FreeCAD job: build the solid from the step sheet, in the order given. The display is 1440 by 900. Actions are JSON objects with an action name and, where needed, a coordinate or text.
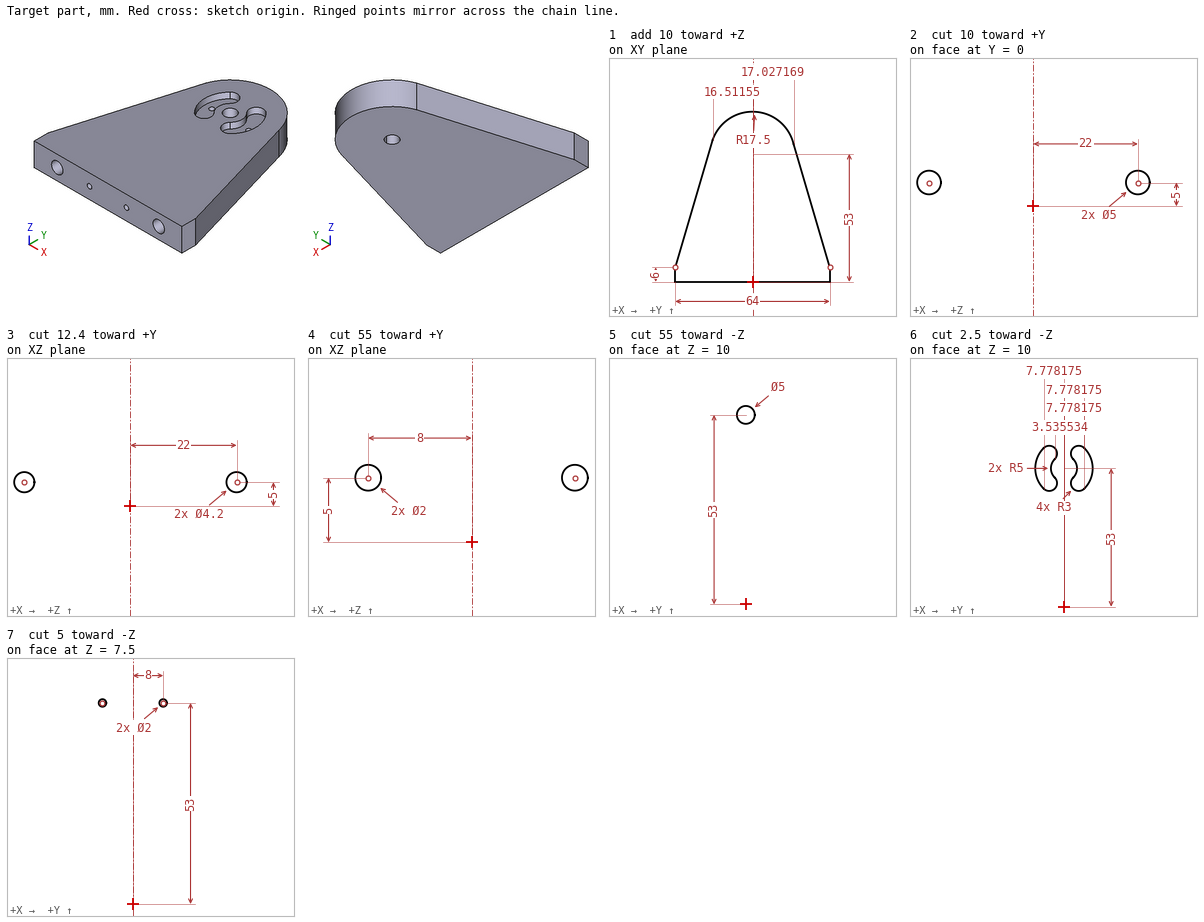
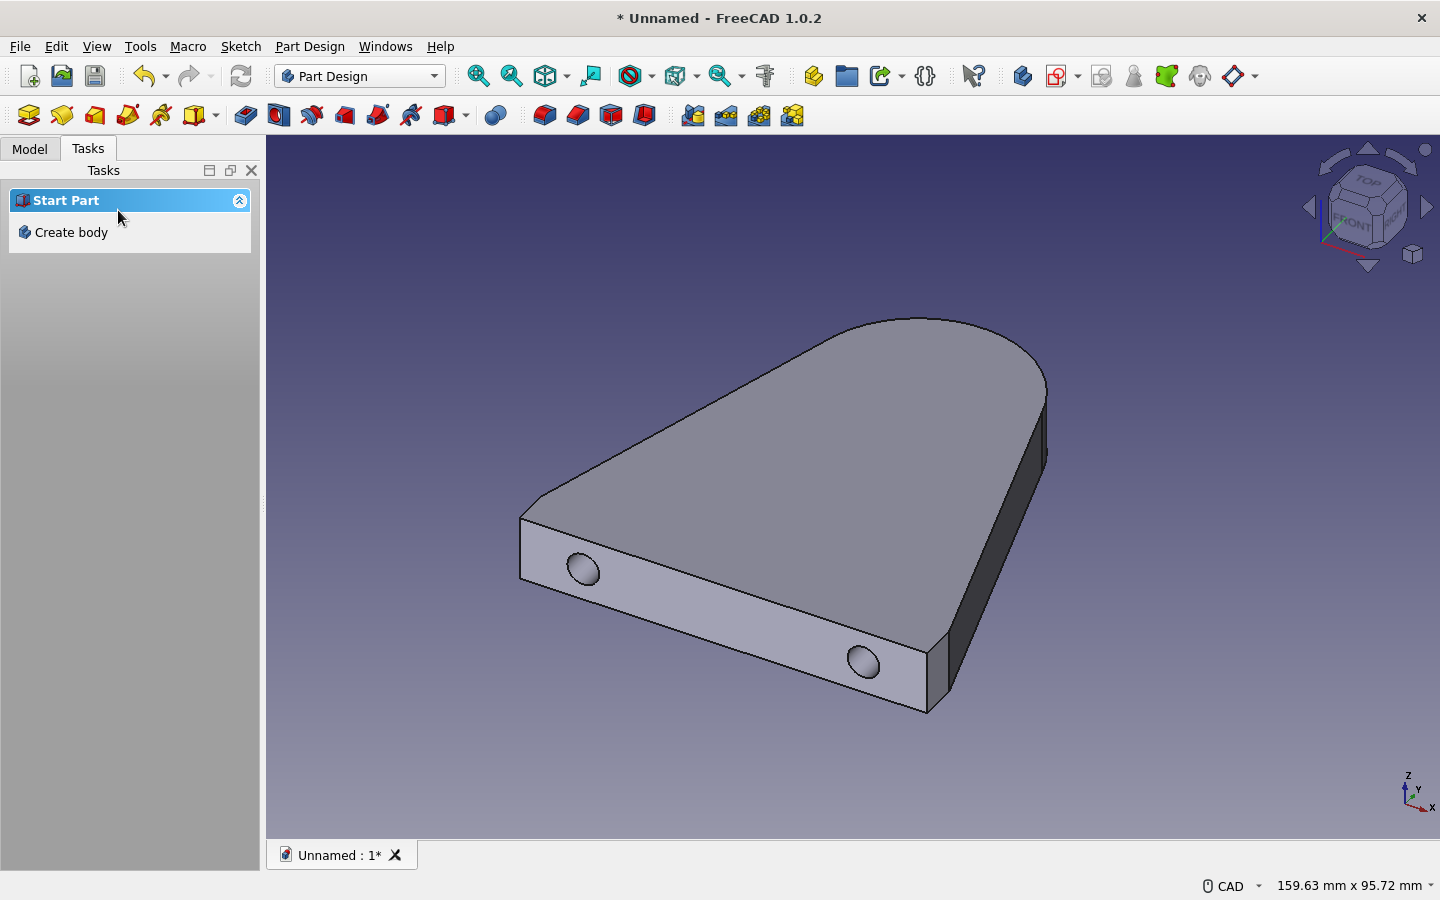
{"action": "left_click", "coordinate": [1056, 76]}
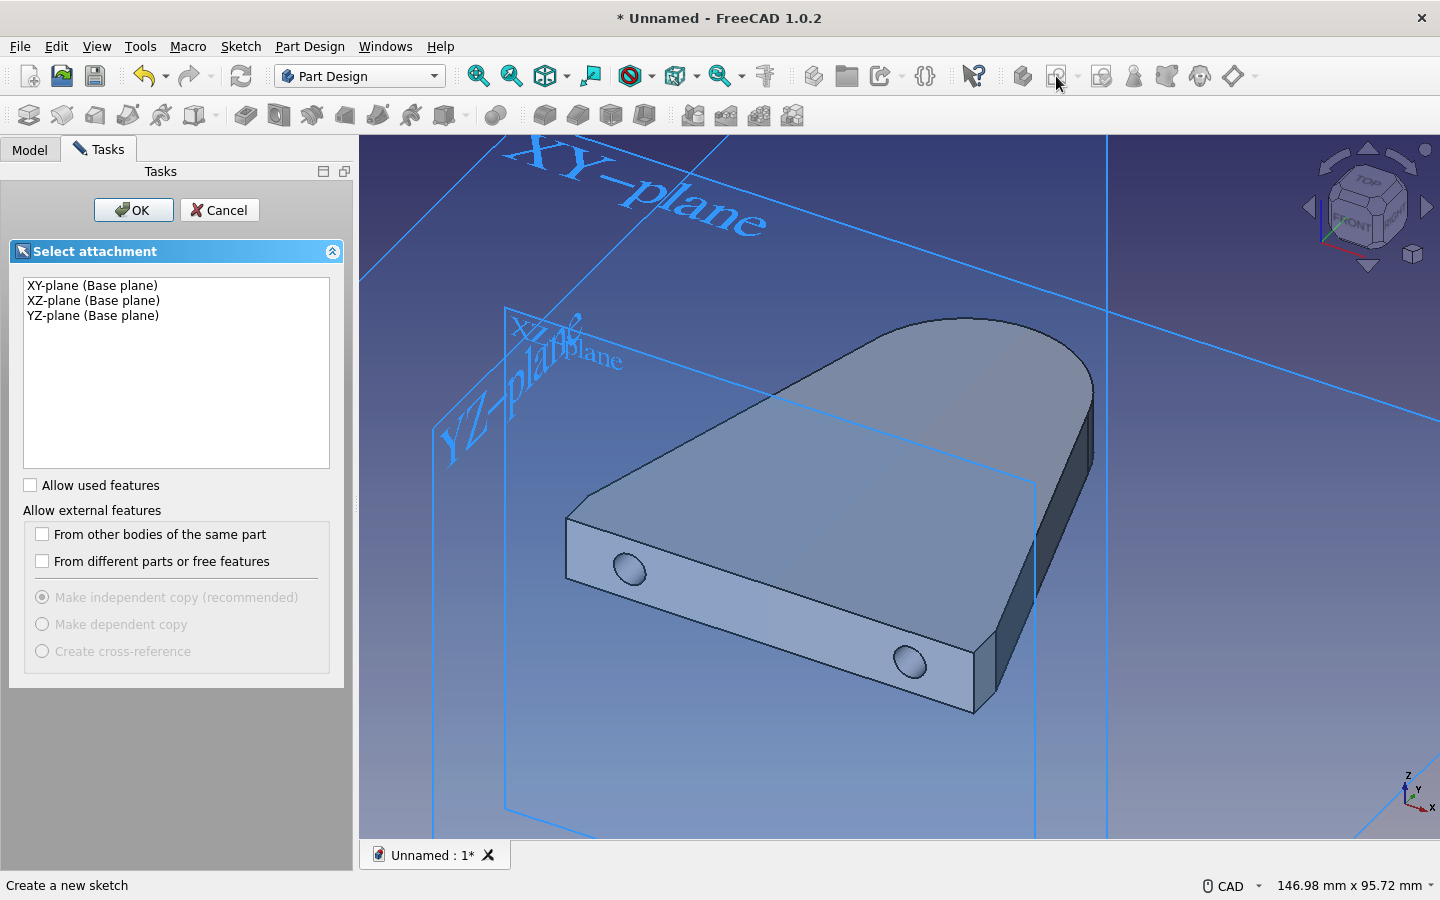
{"action": "left_click", "coordinate": [84, 300]}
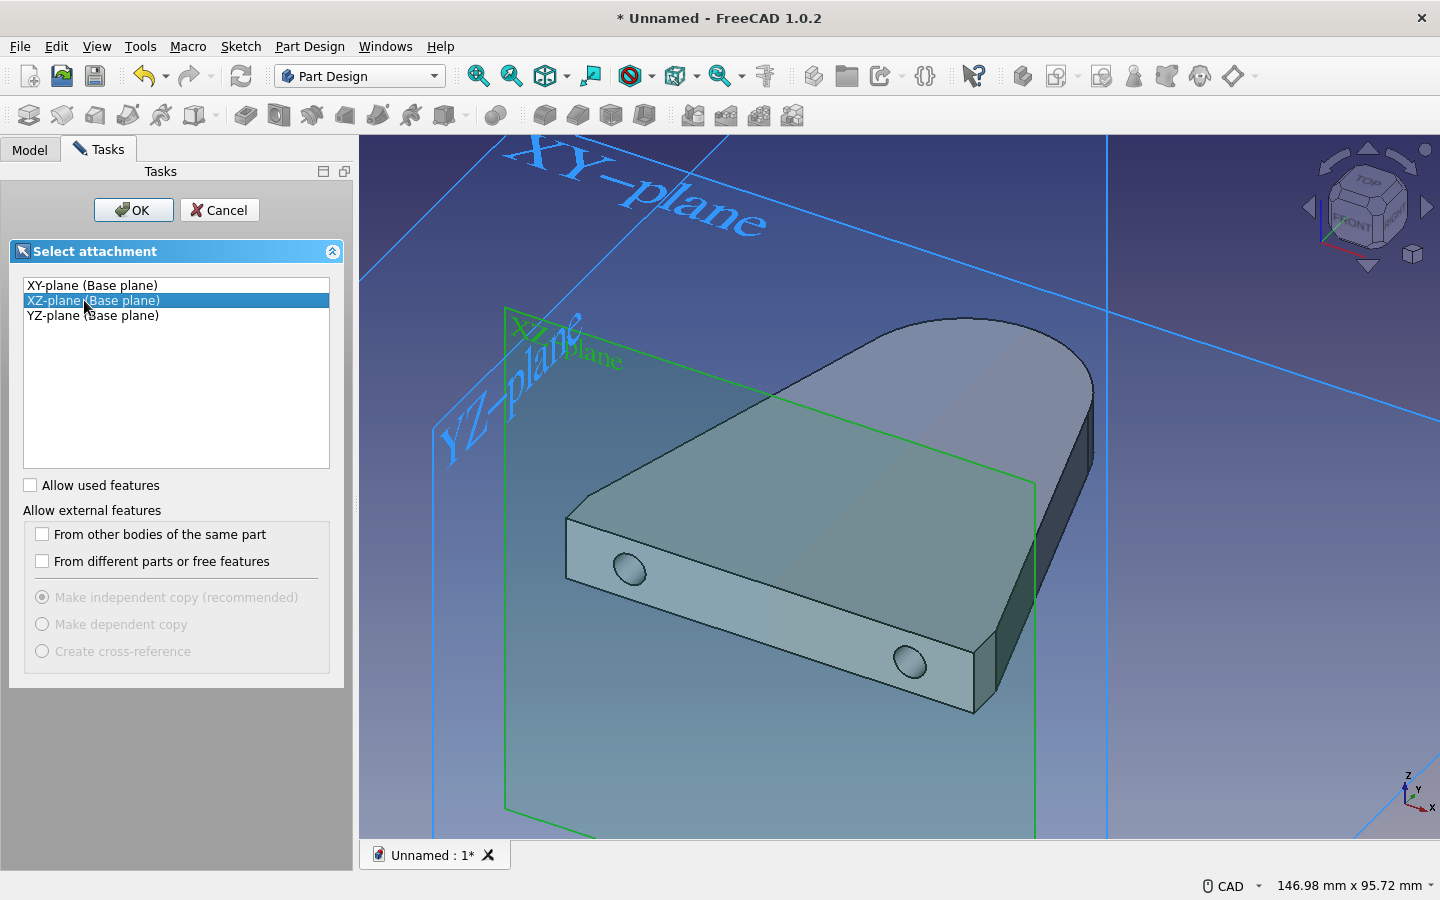
{"action": "left_click", "coordinate": [134, 210]}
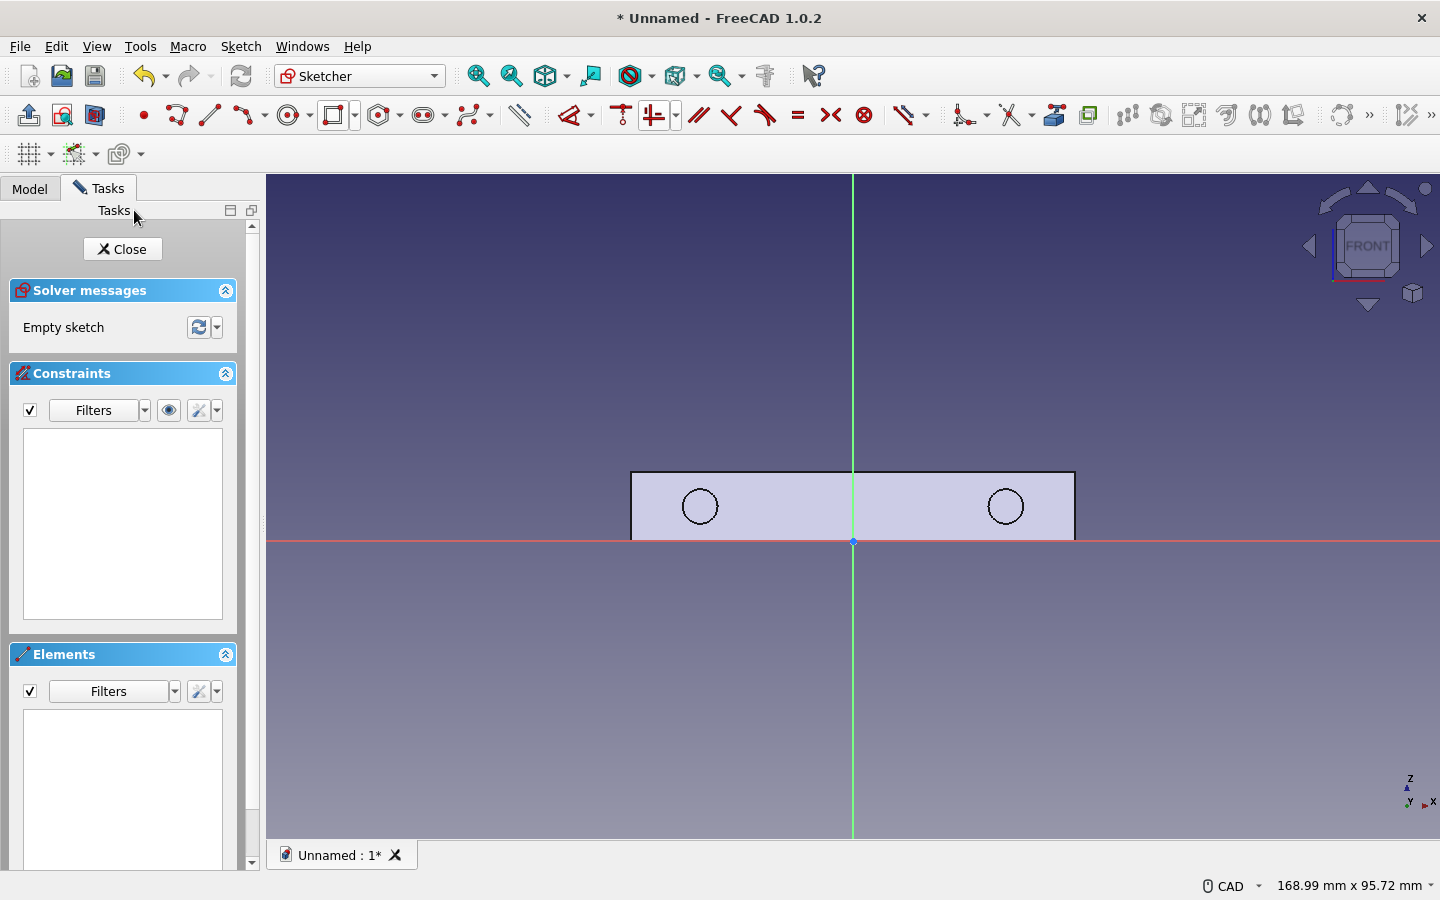
{"action": "scroll", "coordinate": [909, 525], "scroll_direction": "up", "scroll_amount": 4}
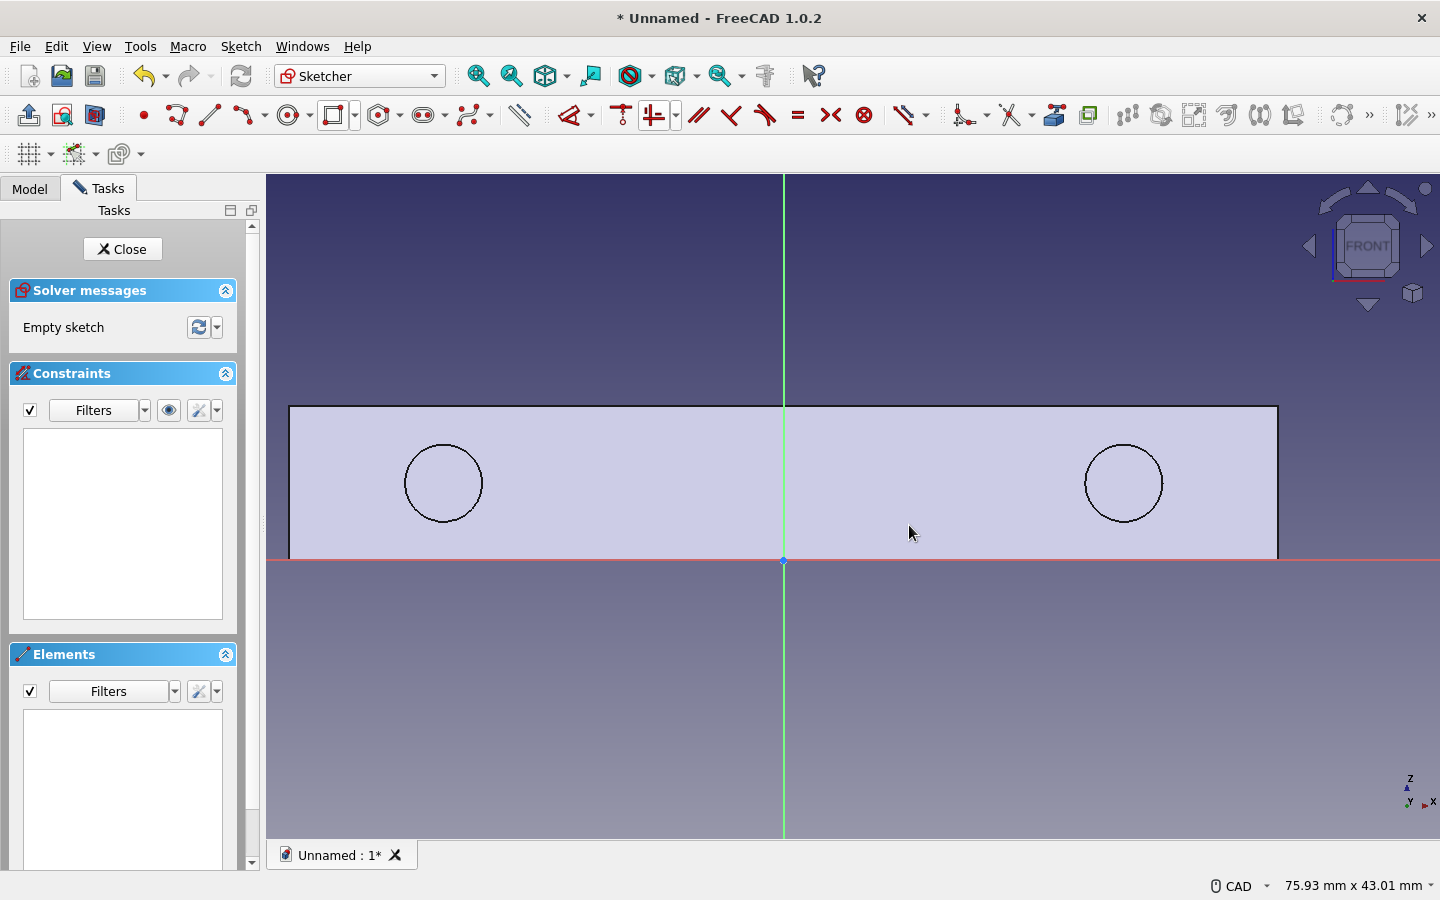
{"action": "left_click", "coordinate": [288, 116]}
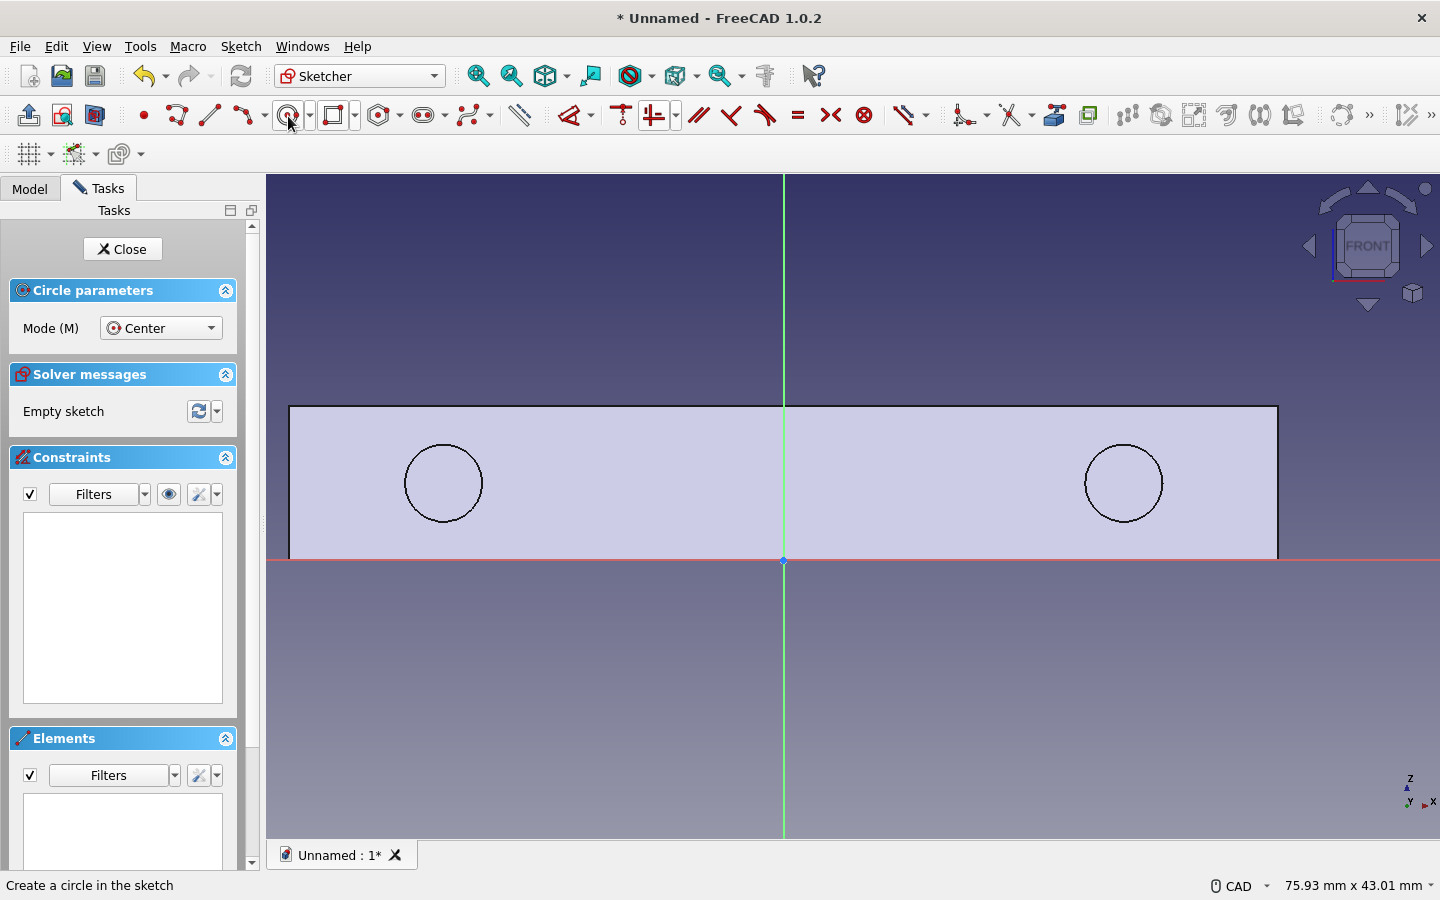
{"action": "left_click", "coordinate": [1124, 483]}
{"action": "mouse_move", "coordinate": [1147, 460]}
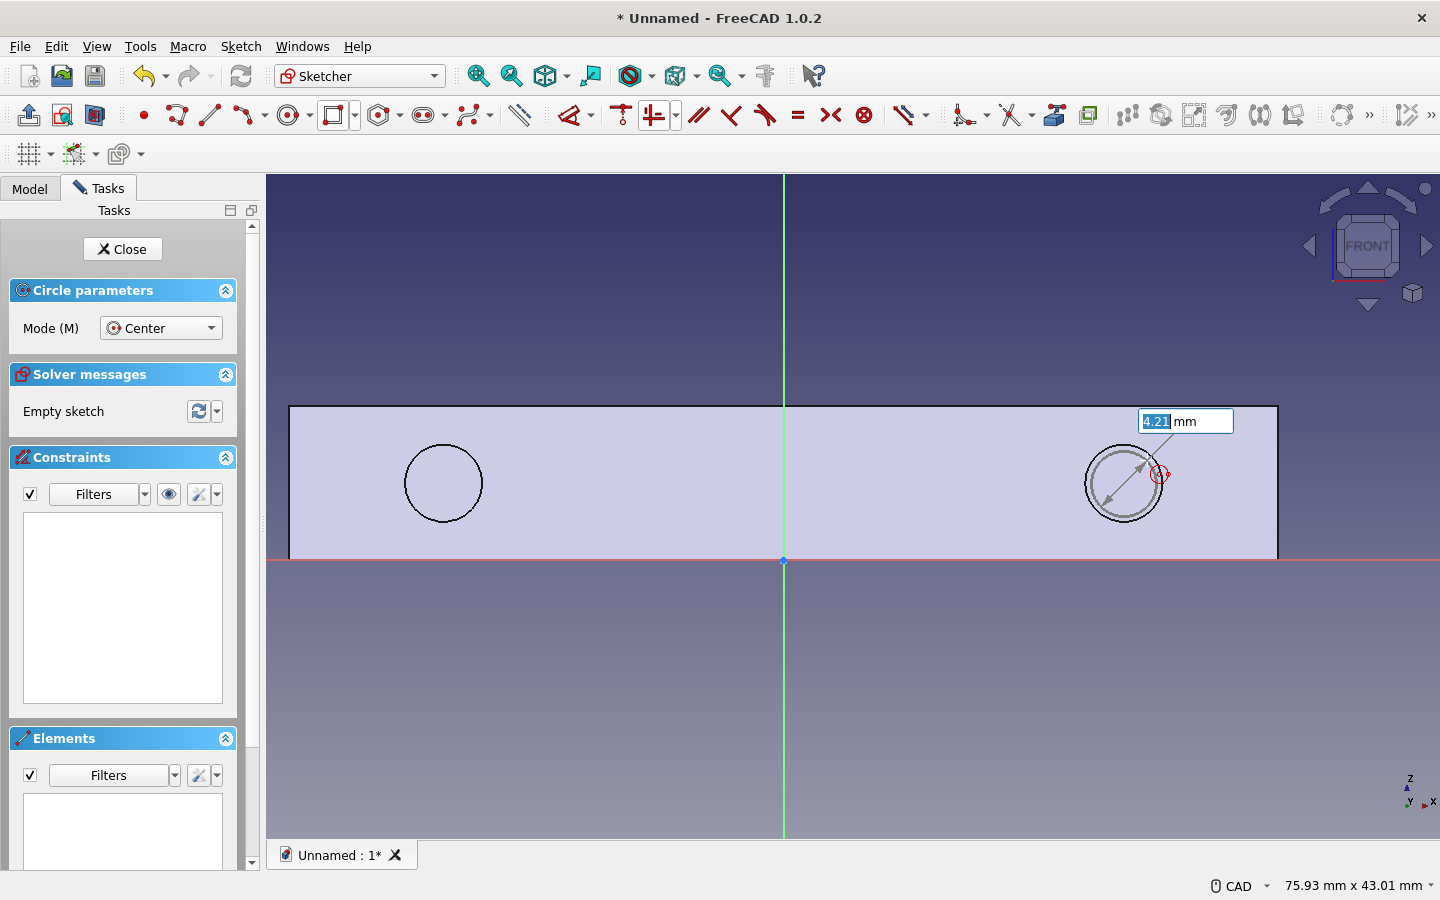
{"action": "type", "text": "4.2"}
{"action": "key", "text": "Return"}